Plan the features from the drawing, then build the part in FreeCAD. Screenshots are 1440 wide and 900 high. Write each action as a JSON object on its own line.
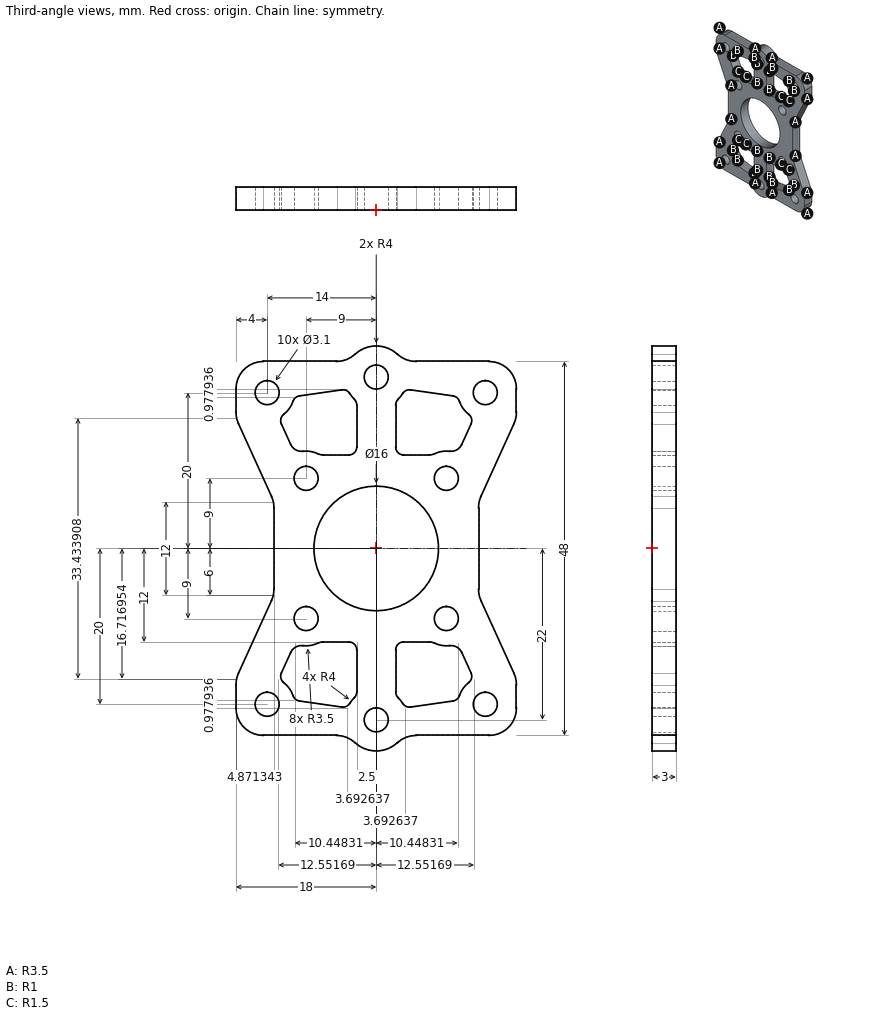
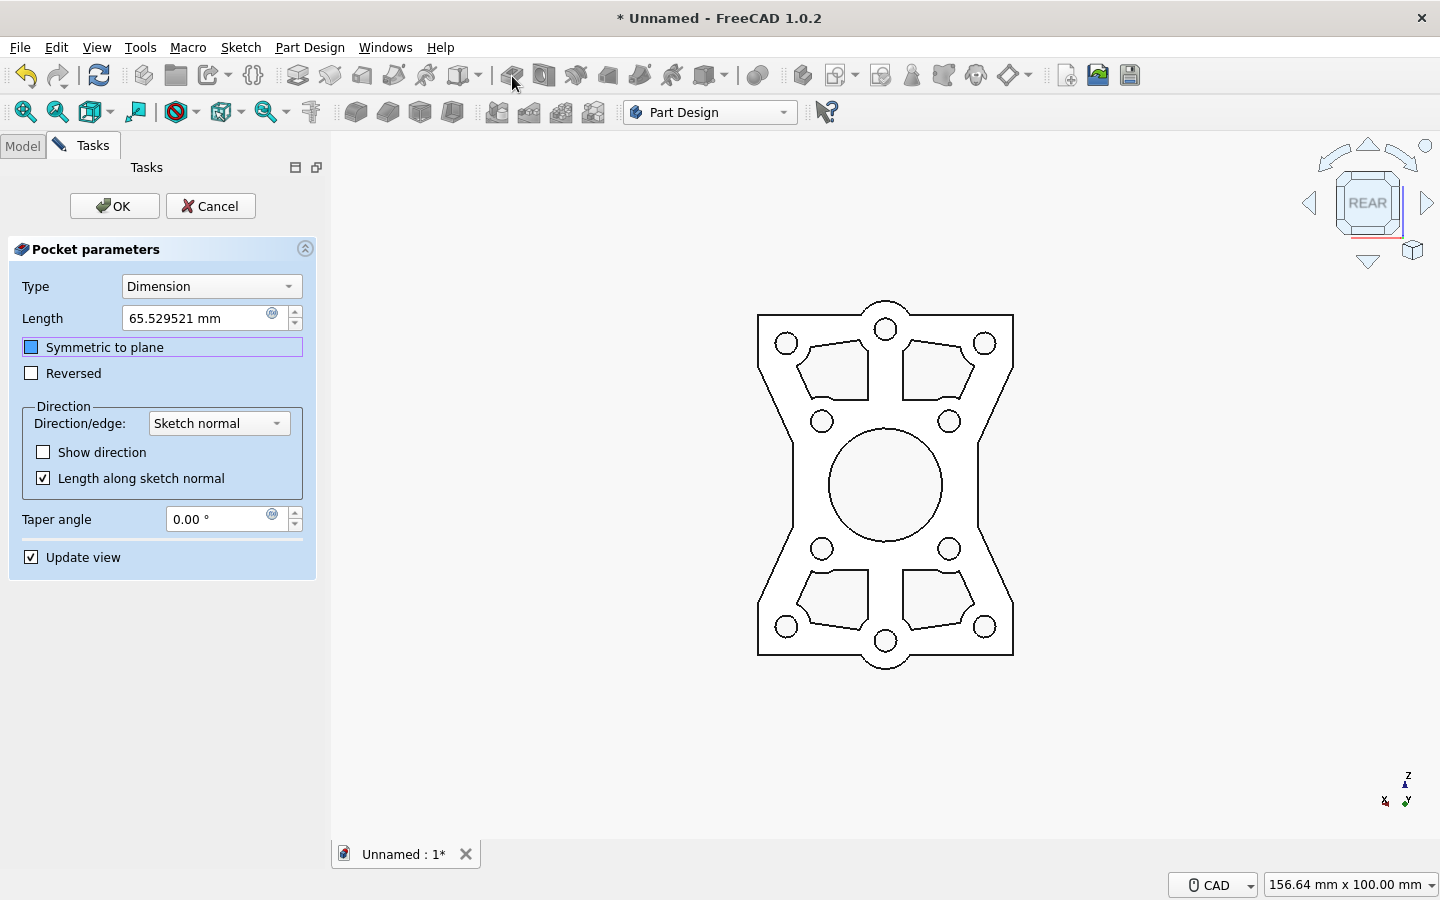
{"action": "left_click", "coordinate": [30, 347]}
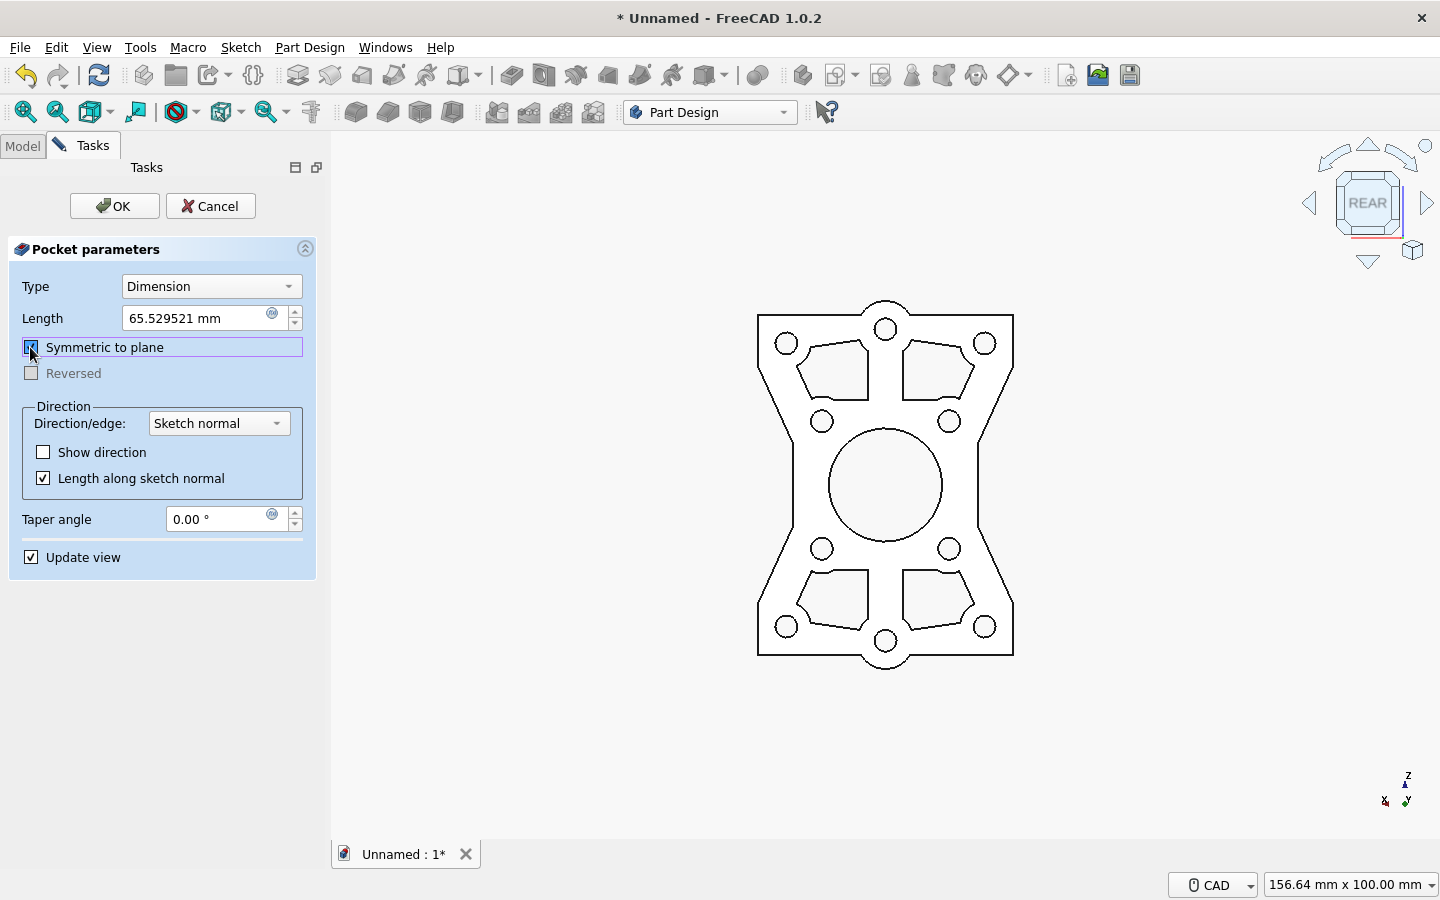
{"action": "left_click", "coordinate": [115, 206]}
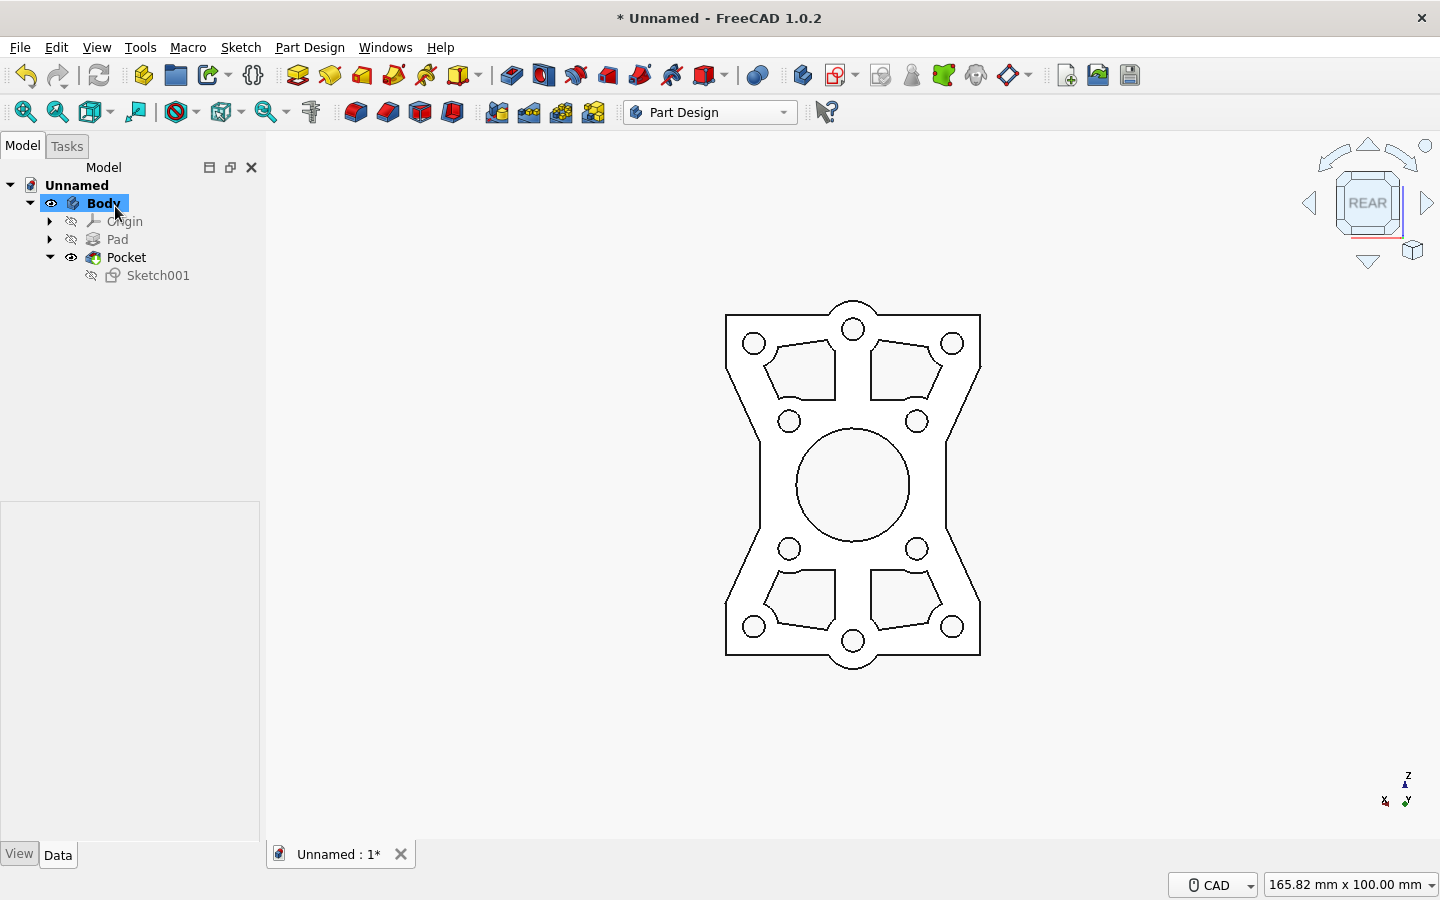
{"action": "scroll", "coordinate": [760, 442], "scroll_direction": "up", "scroll_amount": 4}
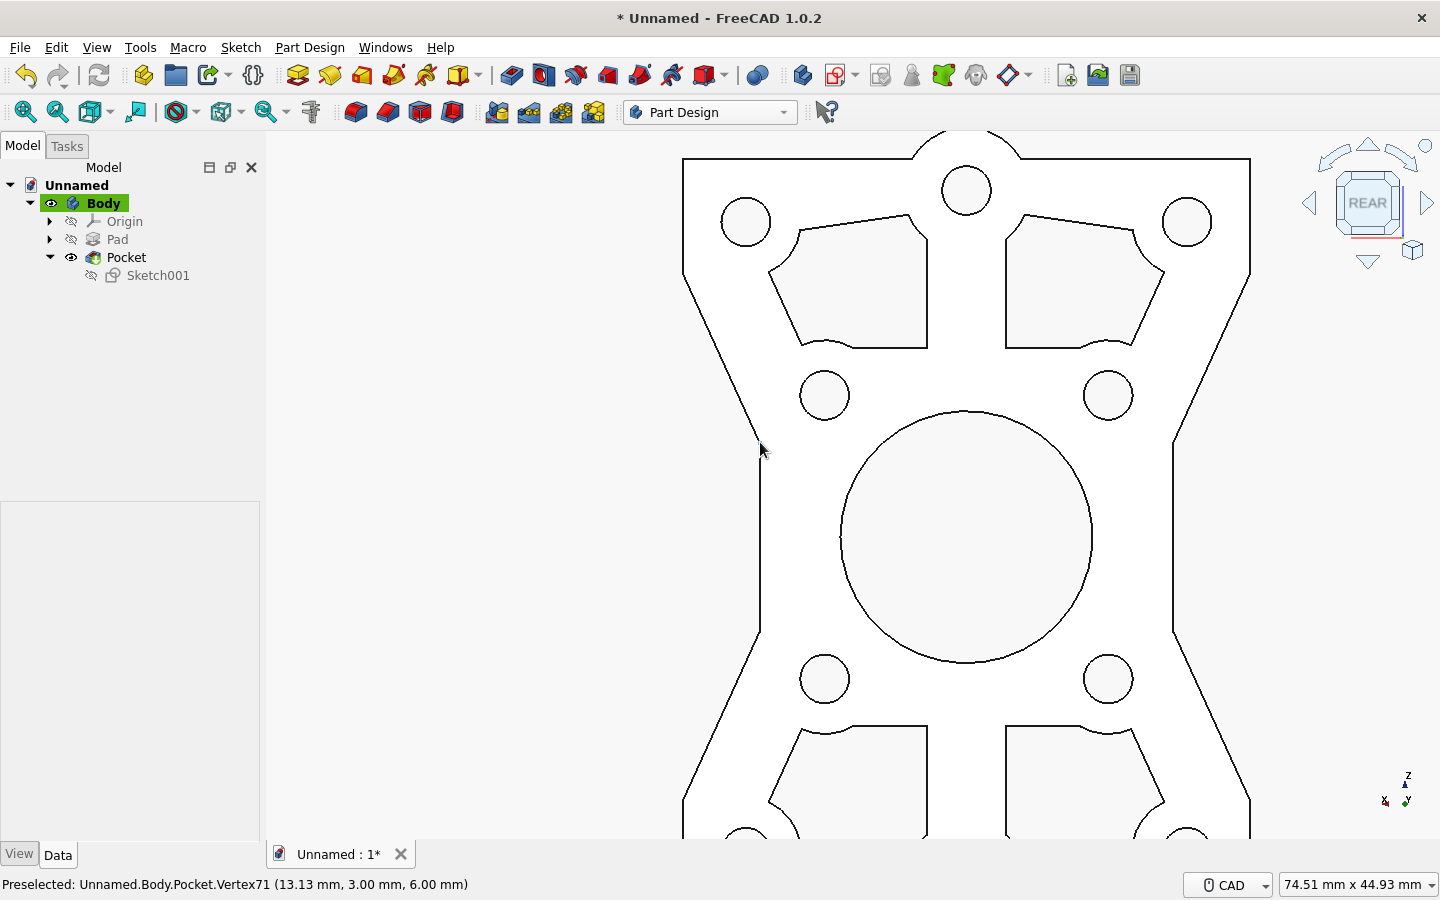
{"action": "left_click", "coordinate": [26, 112]}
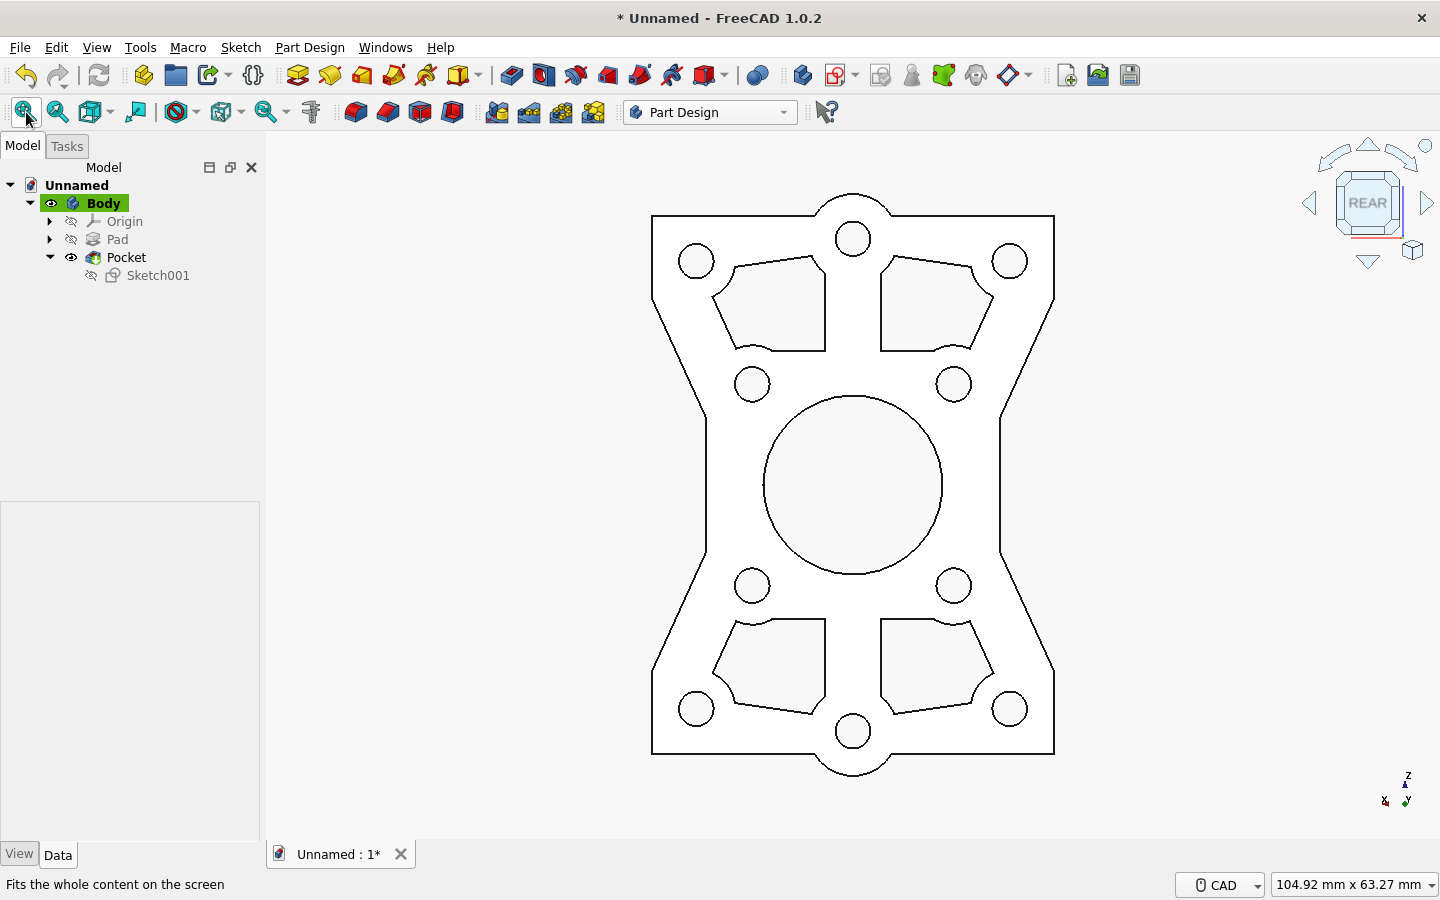
{"action": "key", "text": "0"}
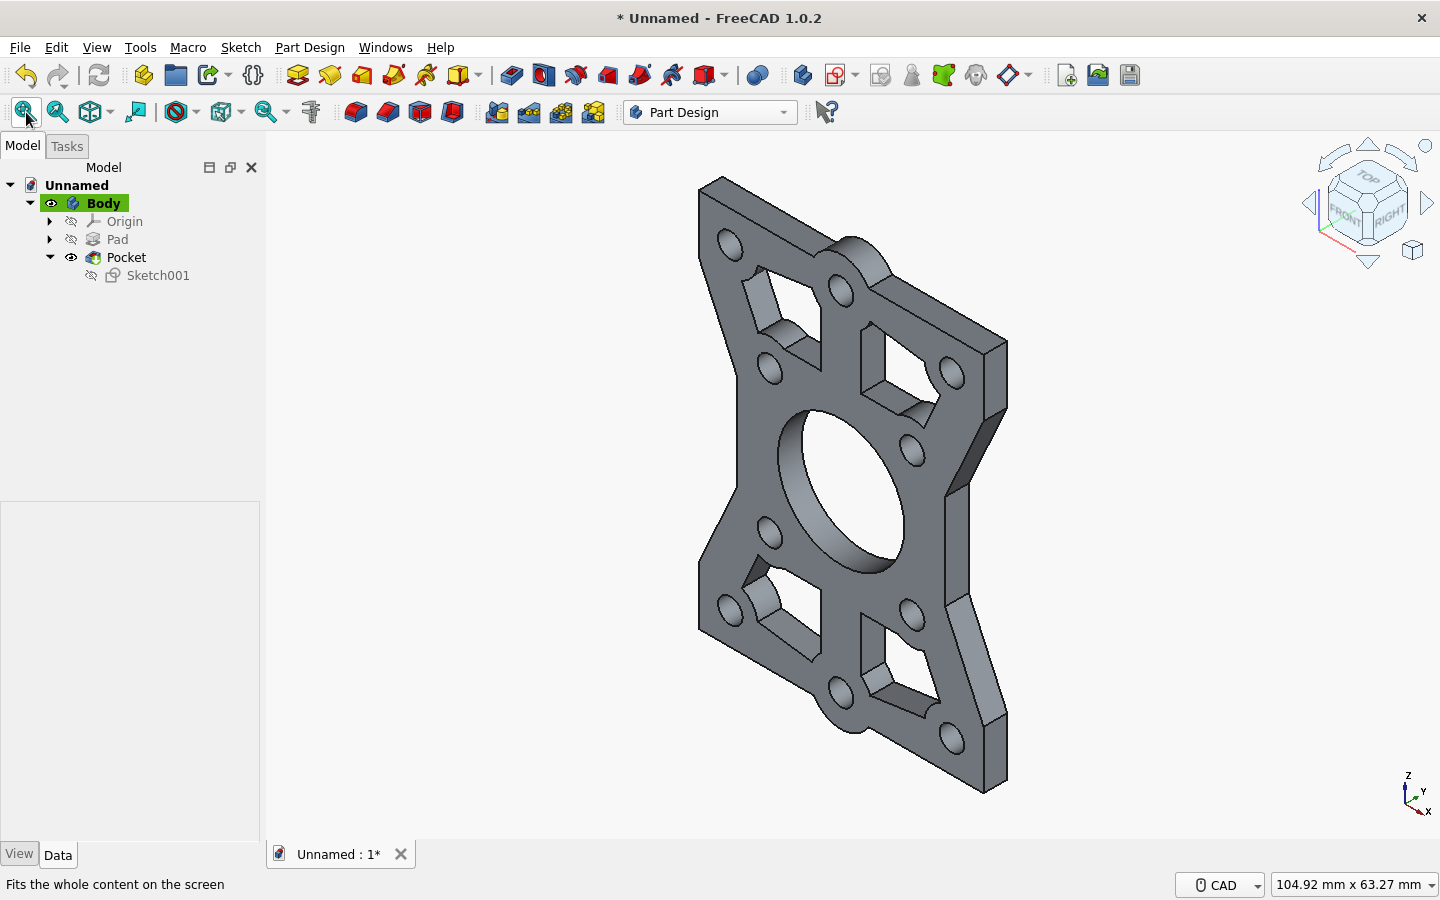
{"action": "left_click", "coordinate": [995, 347]}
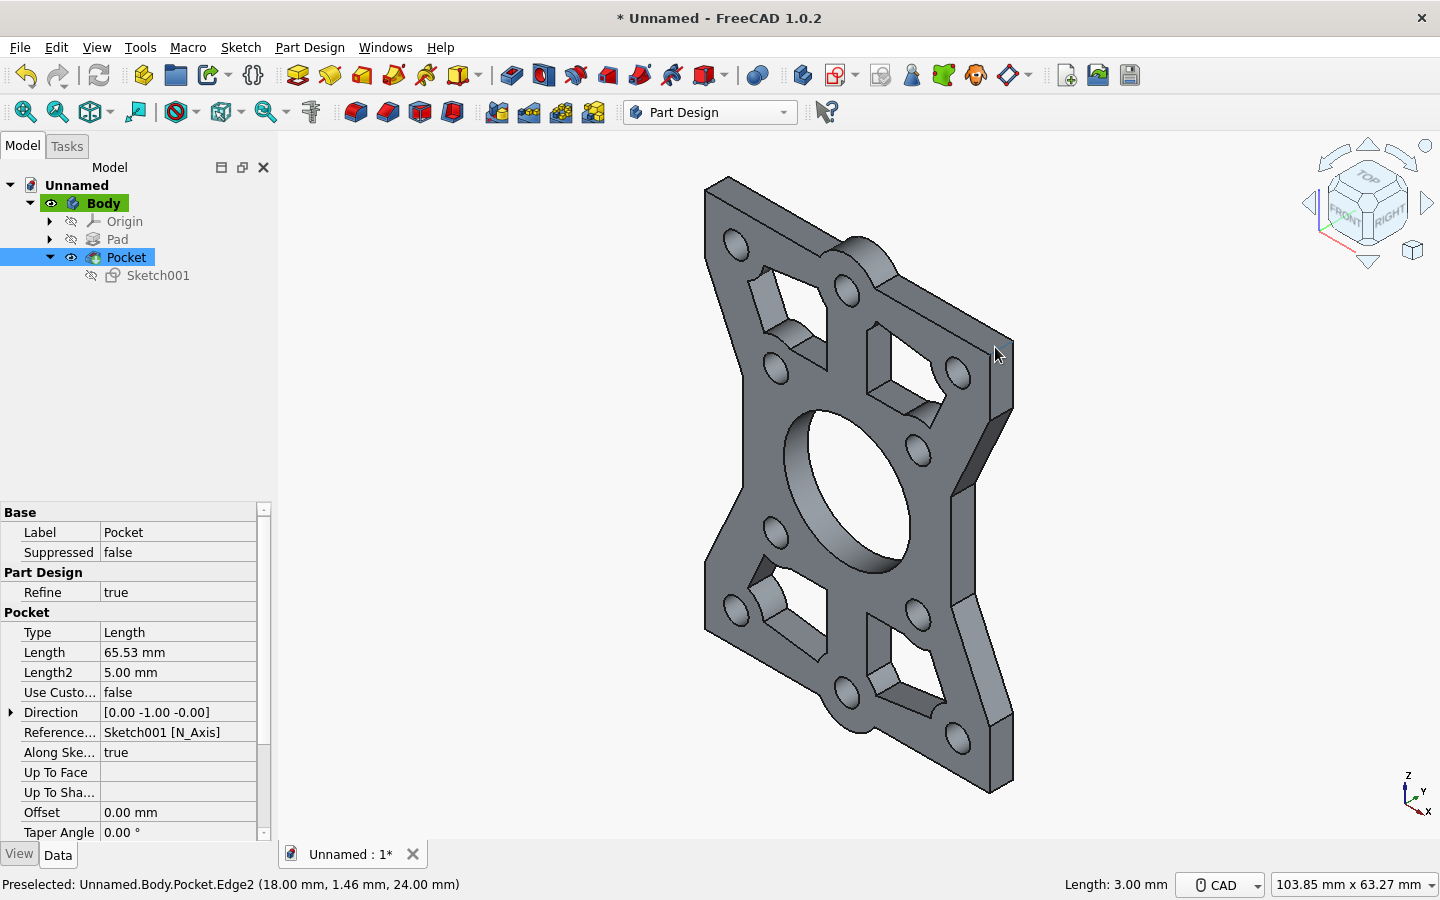
{"action": "key", "text": "2"}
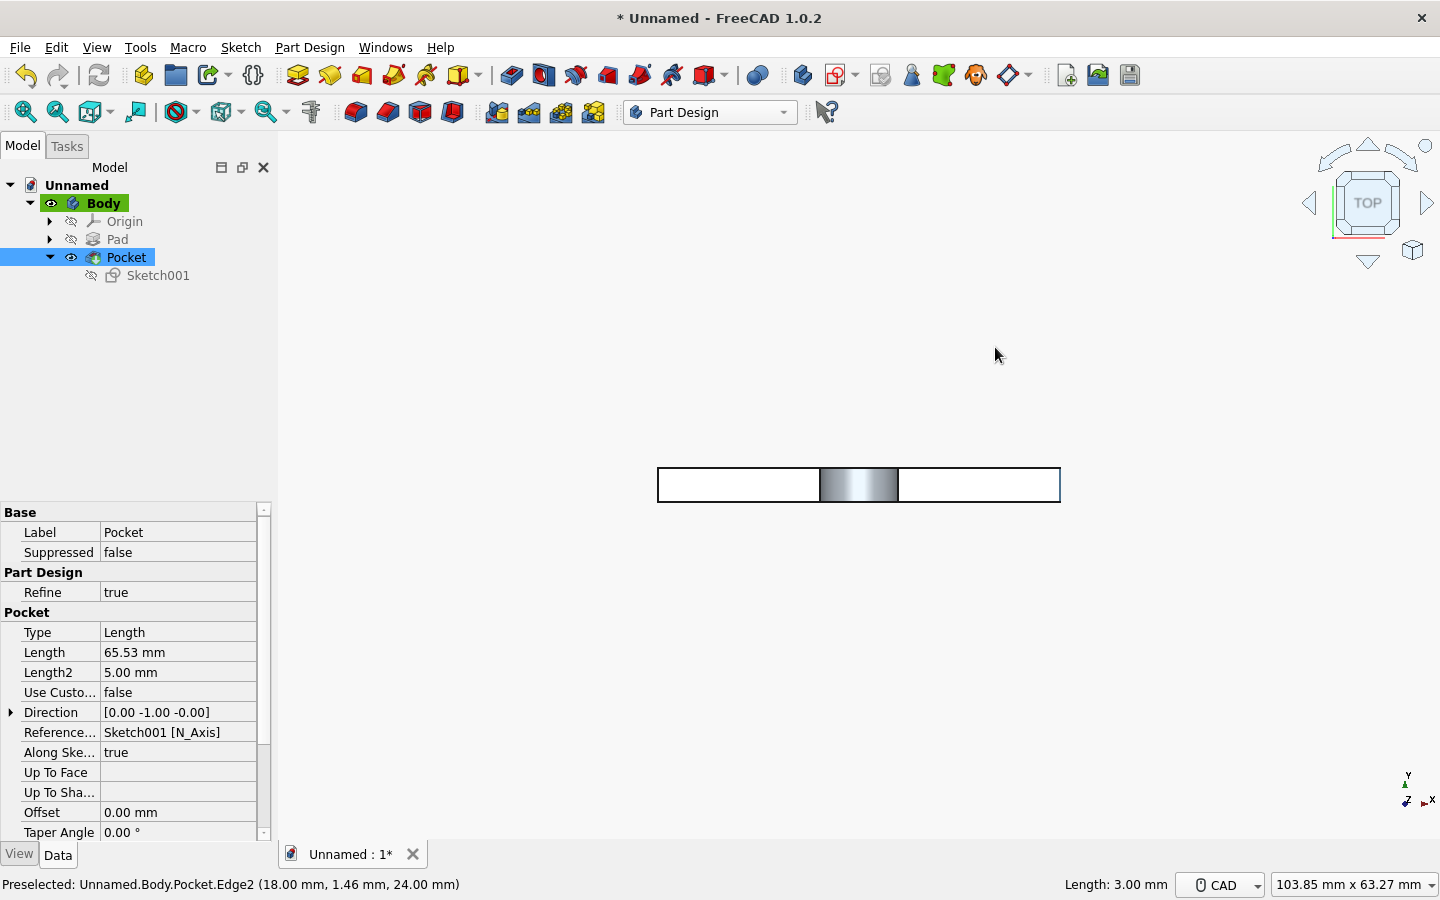
{"action": "left_click", "coordinate": [26, 112]}